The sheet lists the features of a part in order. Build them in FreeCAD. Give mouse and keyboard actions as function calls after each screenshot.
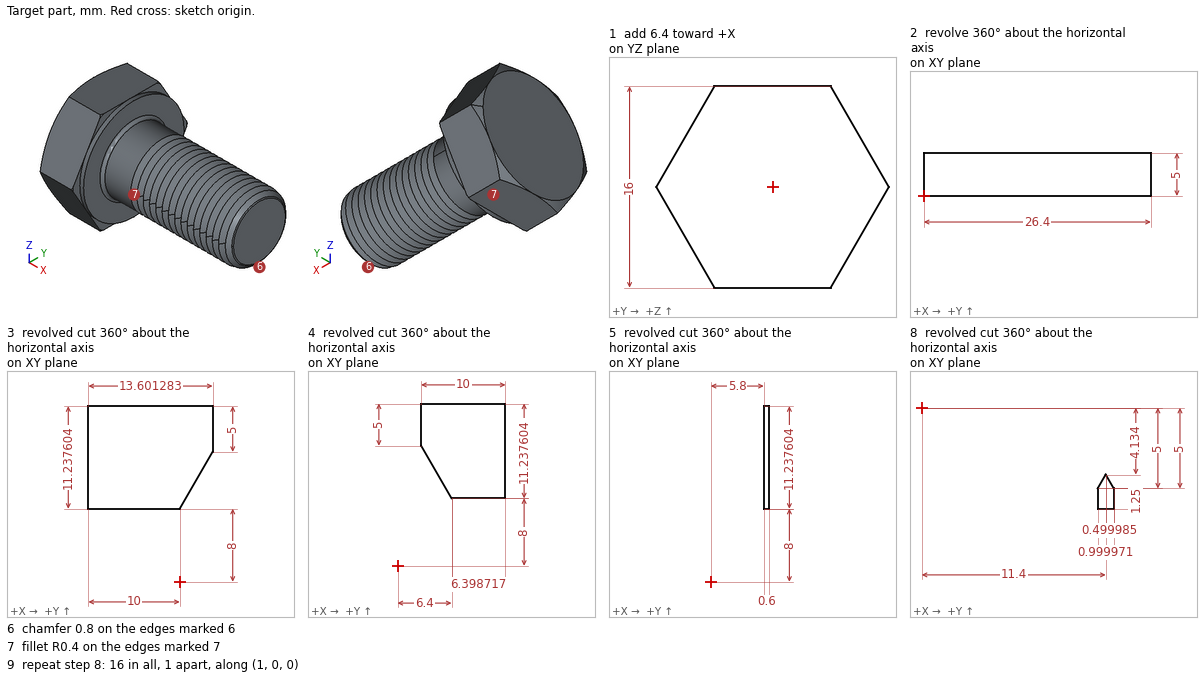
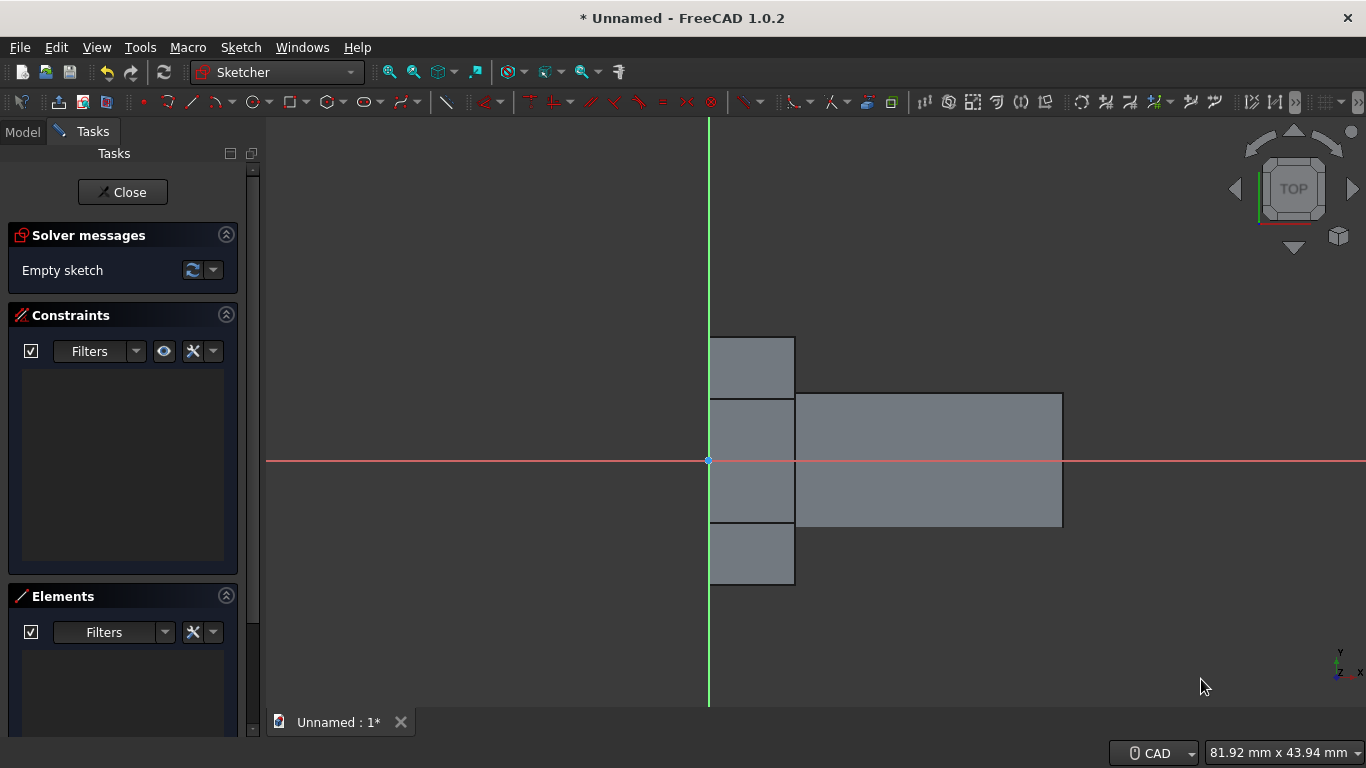
scroll(500, 168, up, 2)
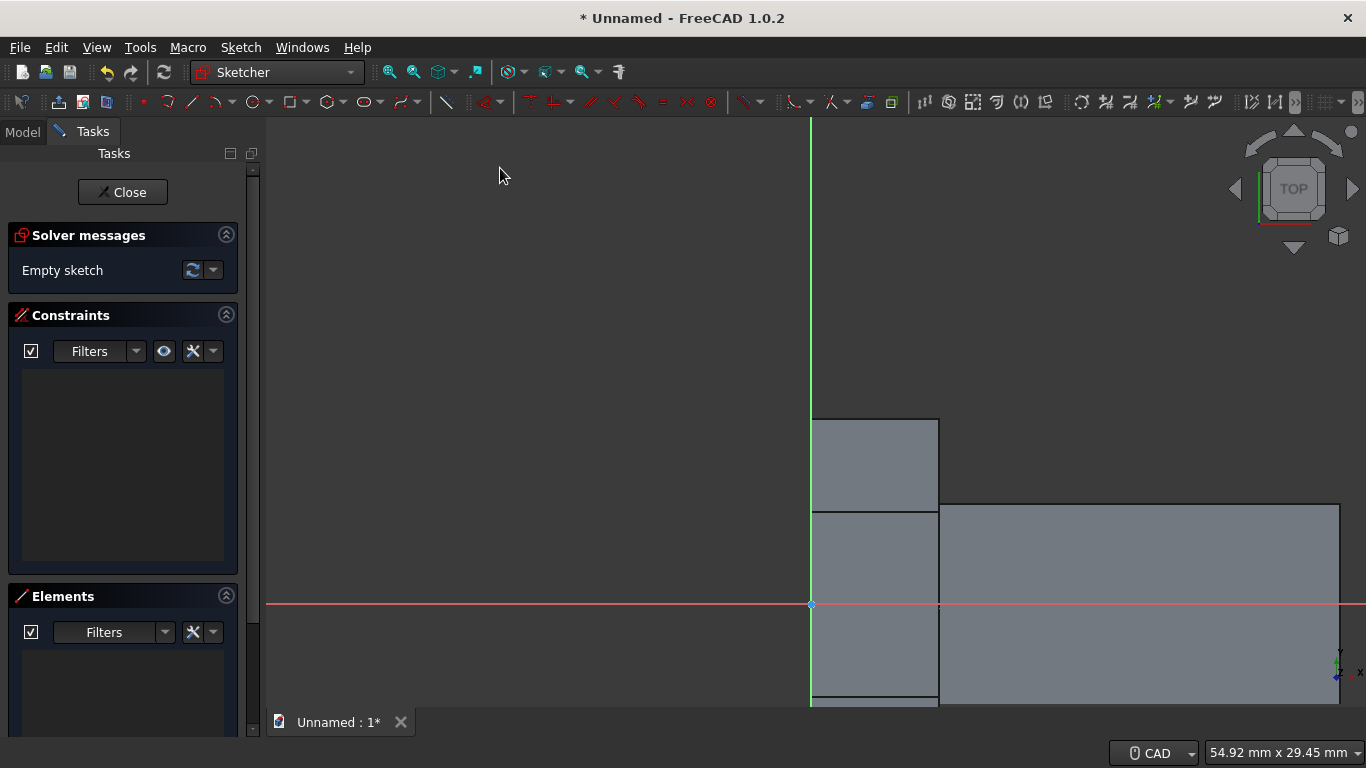
key(g)
key(m)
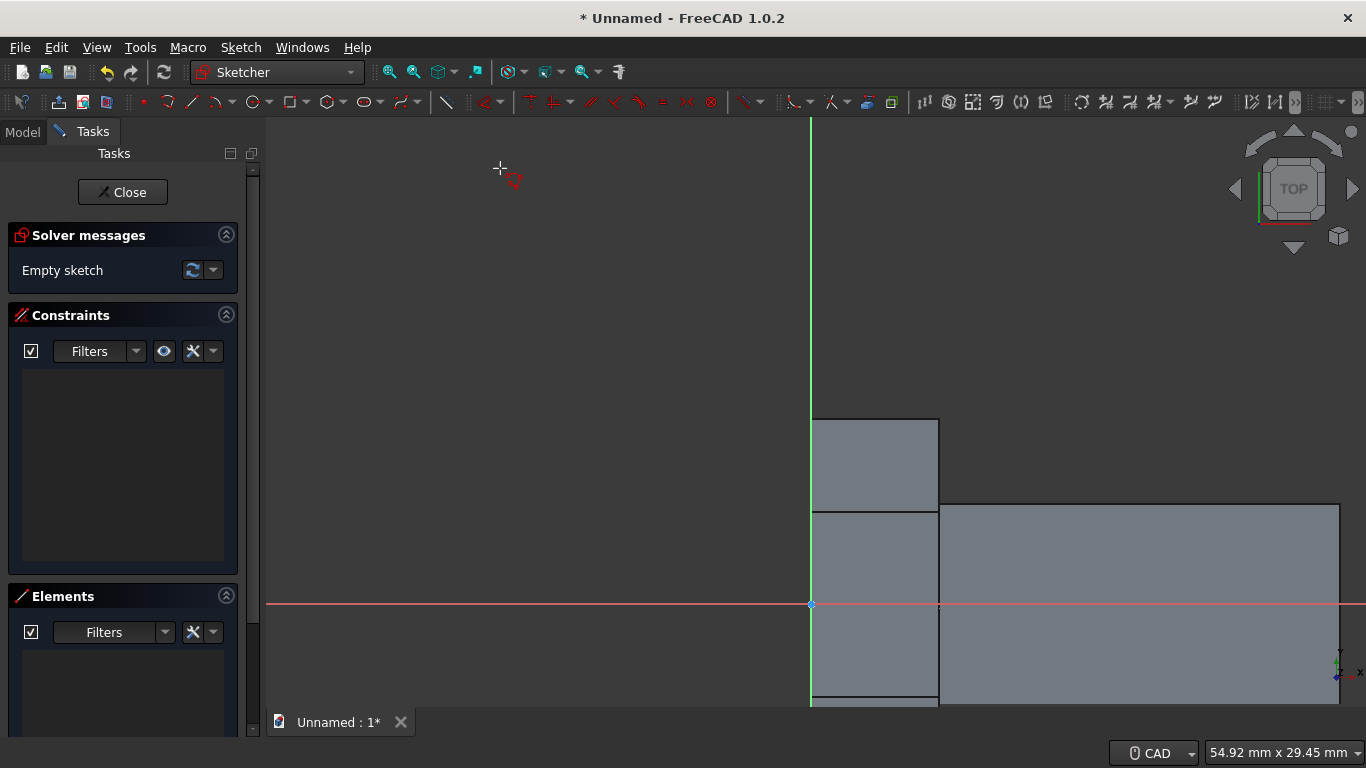
click(811, 444)
click(883, 319)
click(883, 219)
click(611, 219)
click(611, 444)
click(811, 445)
key(Escape)
key(Escape)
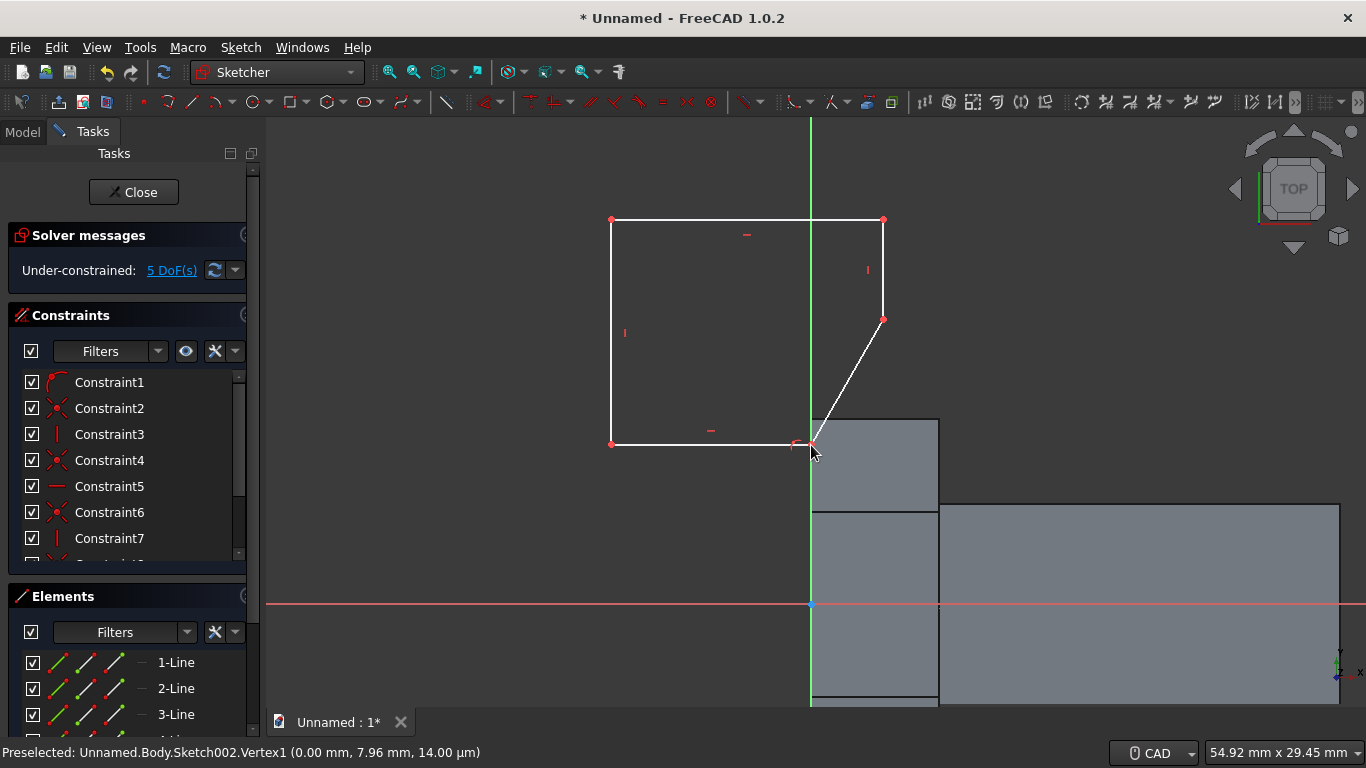
key(d)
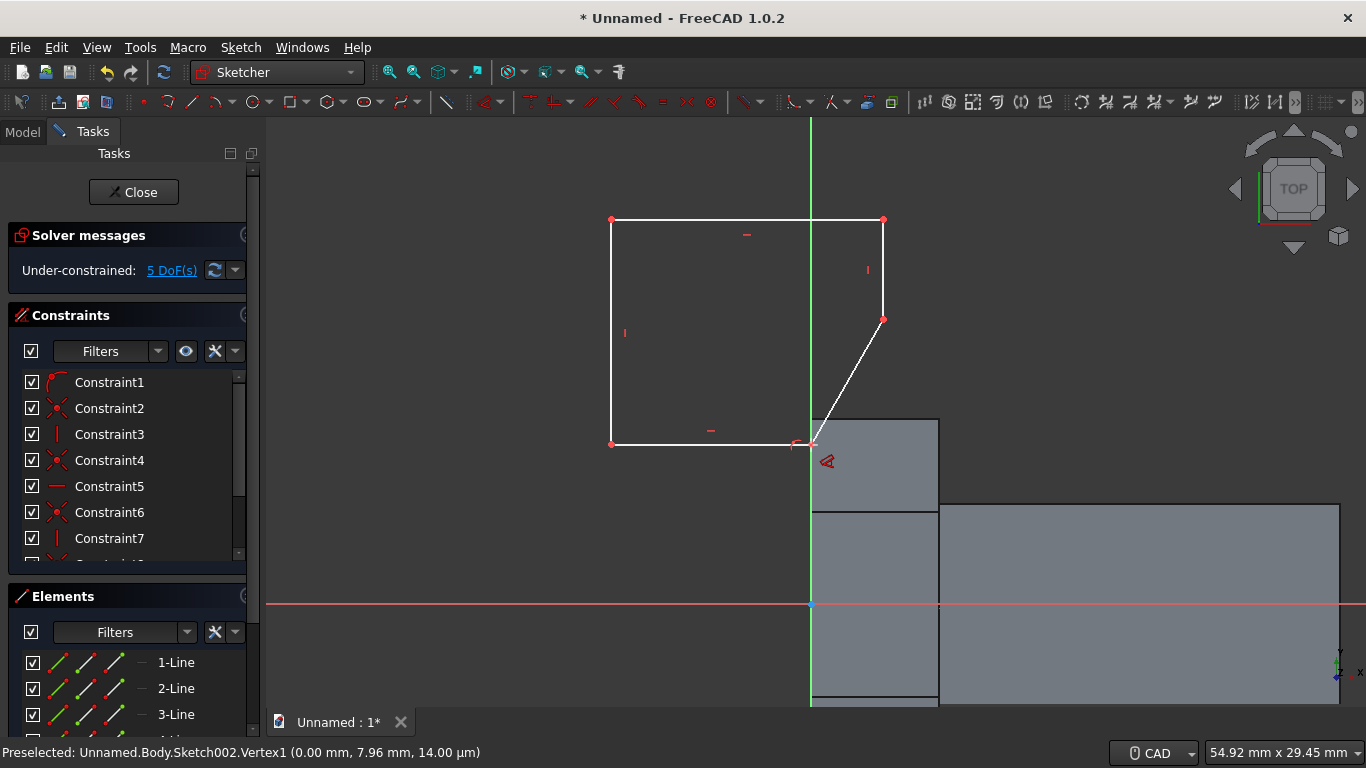
click(883, 290)
click(917, 270)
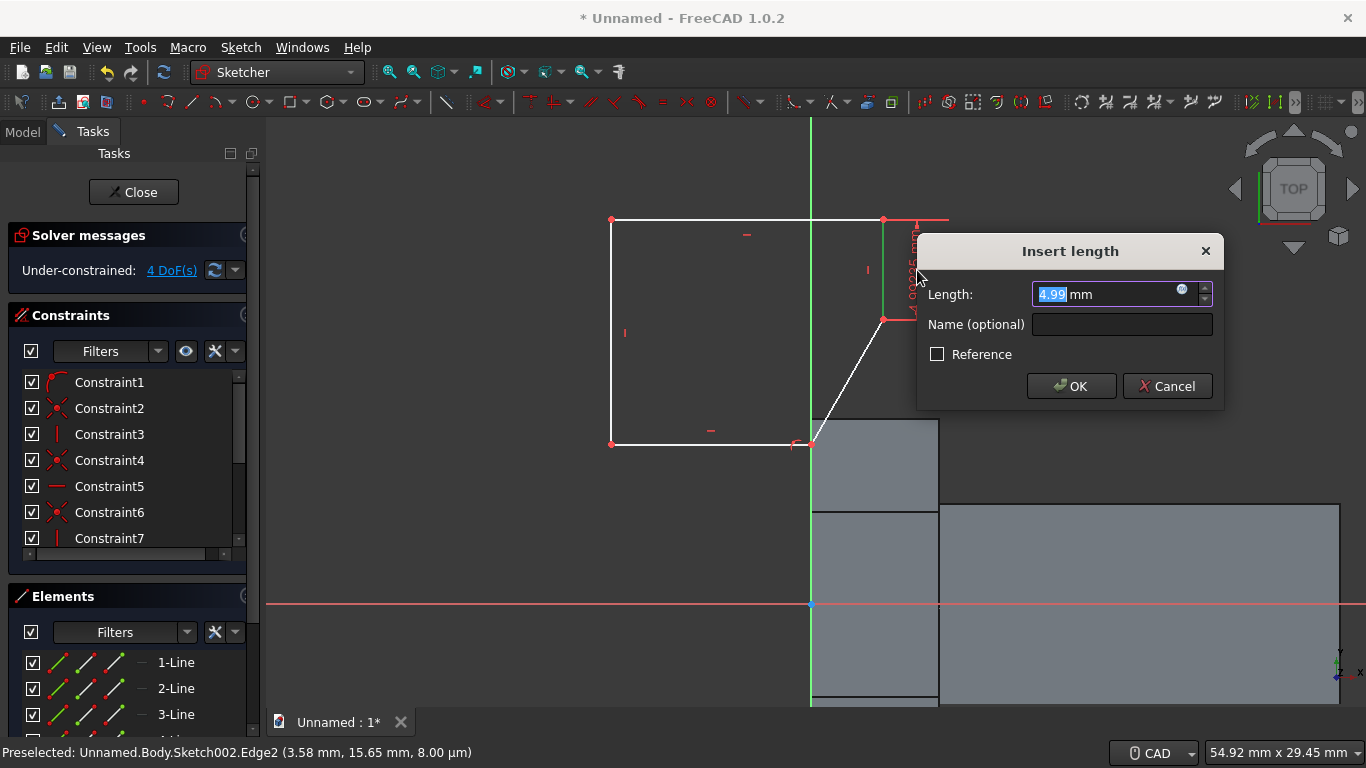
text(5)
key(Return)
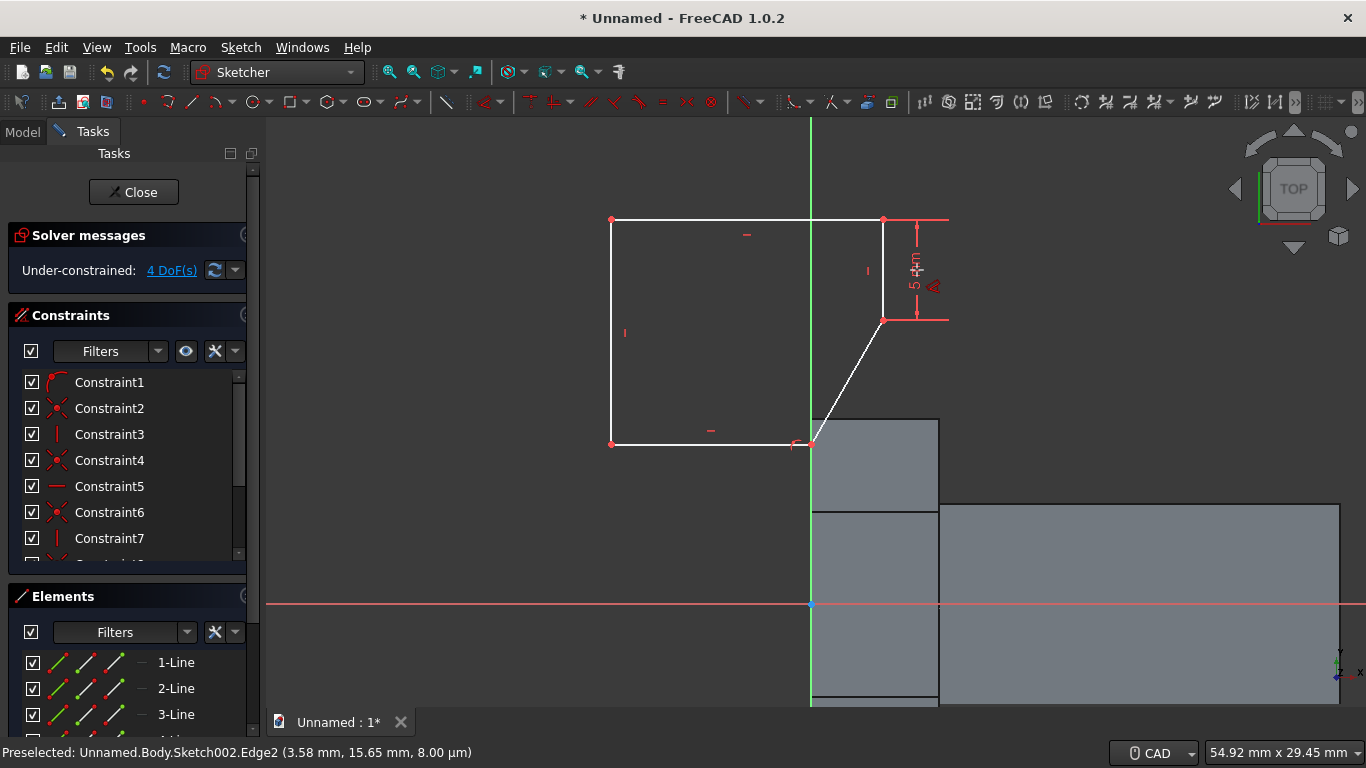
click(671, 445)
click(711, 479)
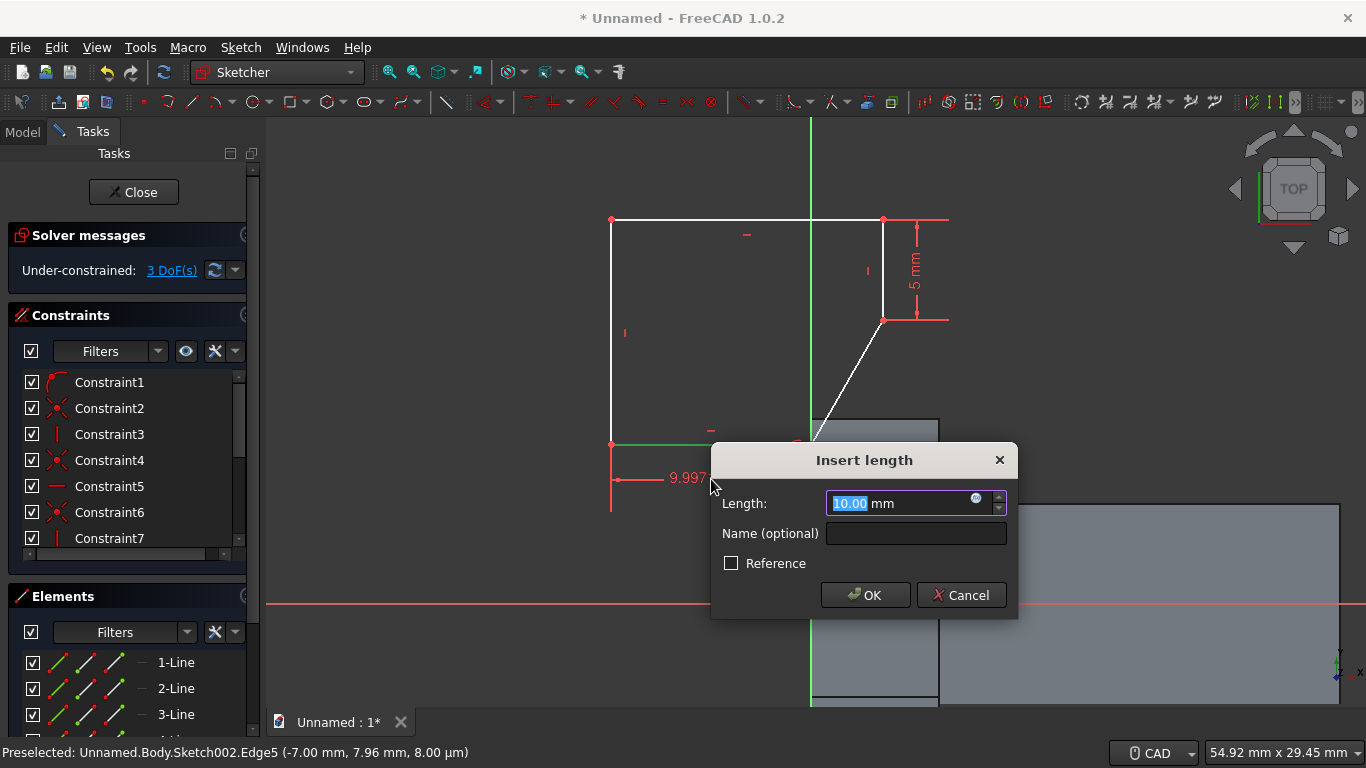
text(10)
key(Return)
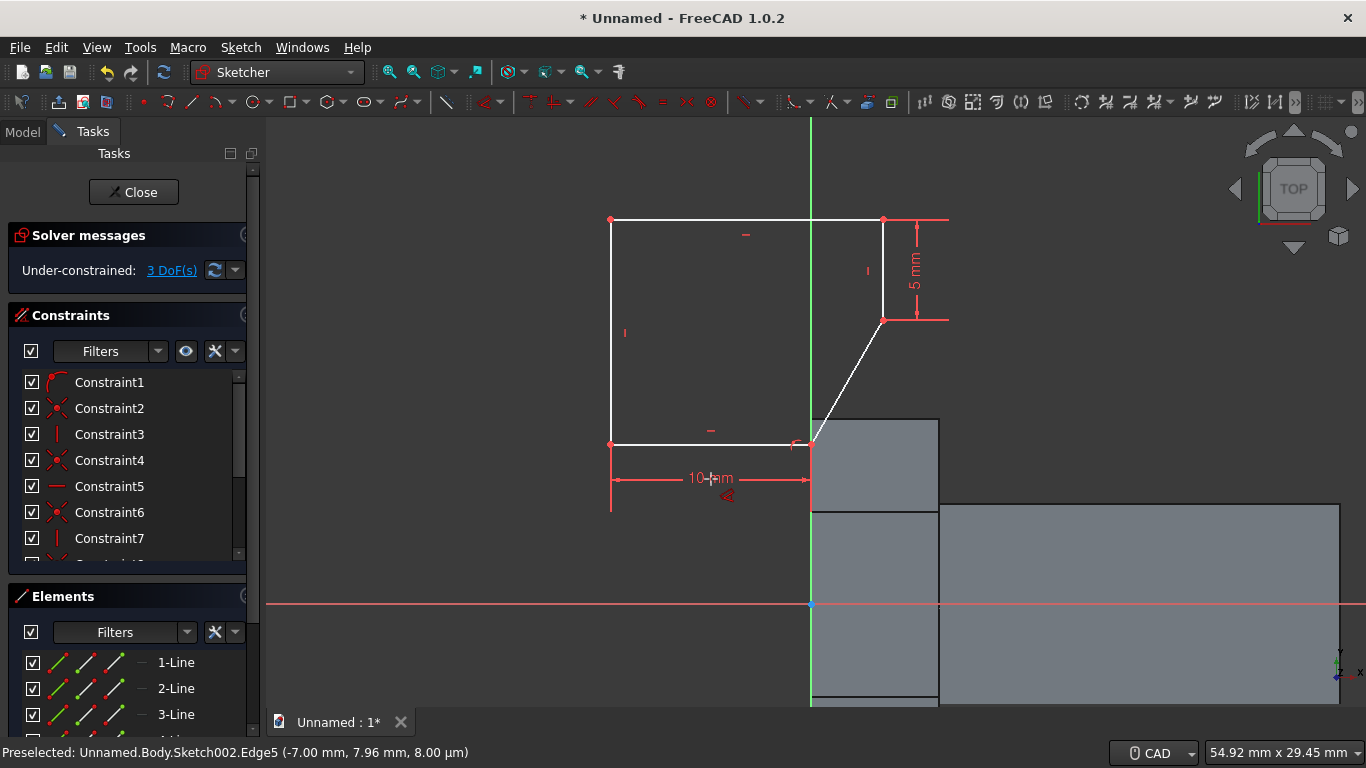
click(811, 445)
click(845, 525)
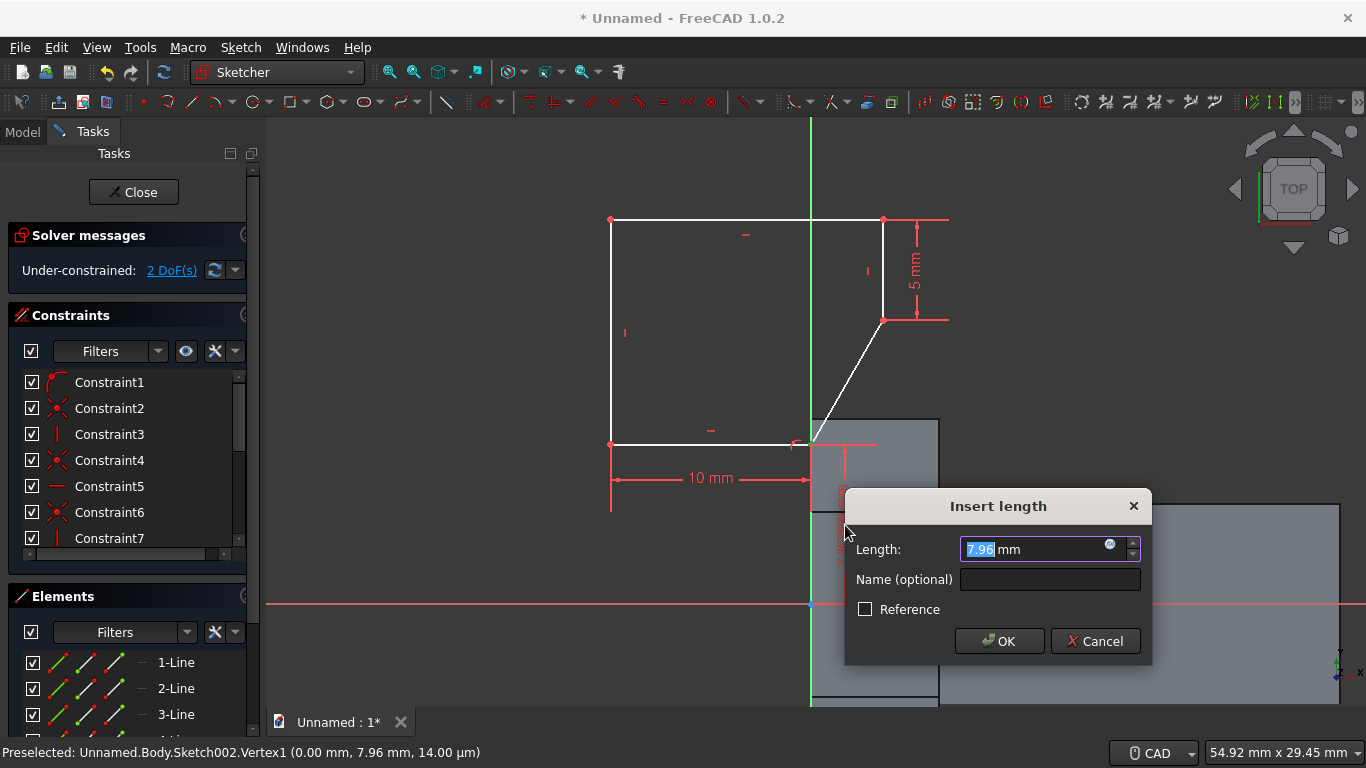
text(8)
key(Return)